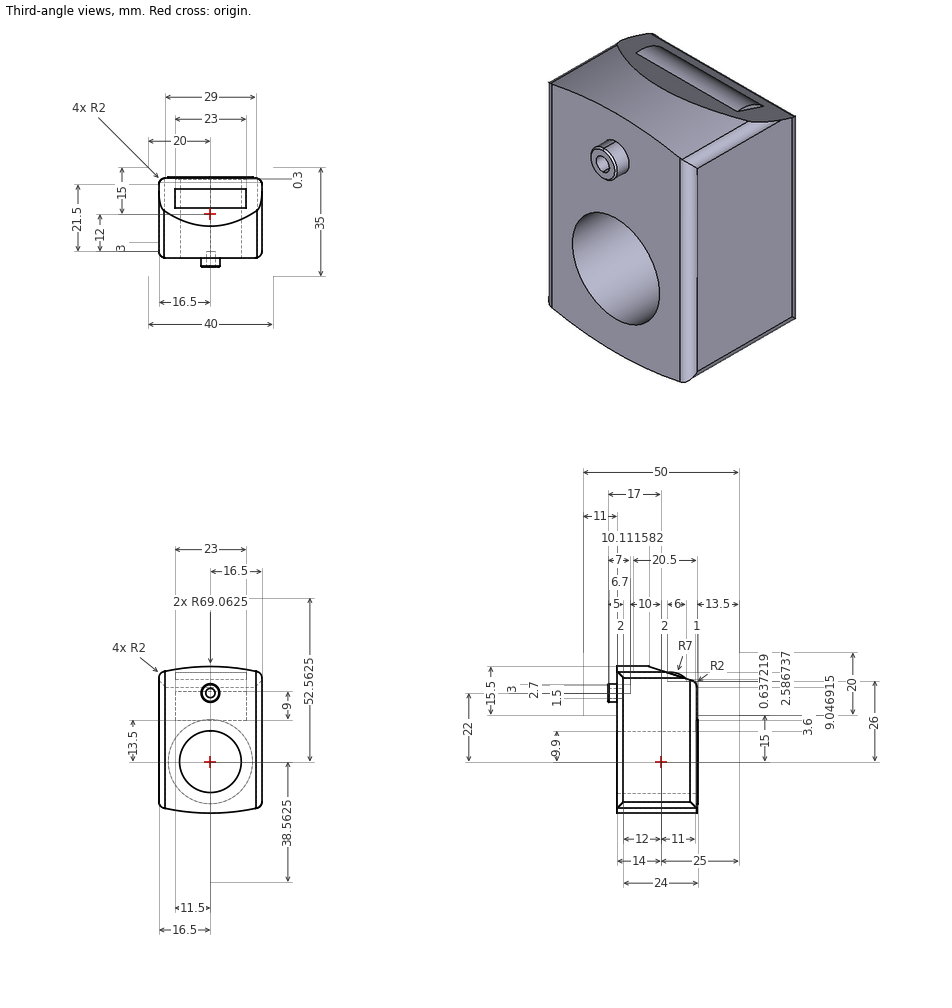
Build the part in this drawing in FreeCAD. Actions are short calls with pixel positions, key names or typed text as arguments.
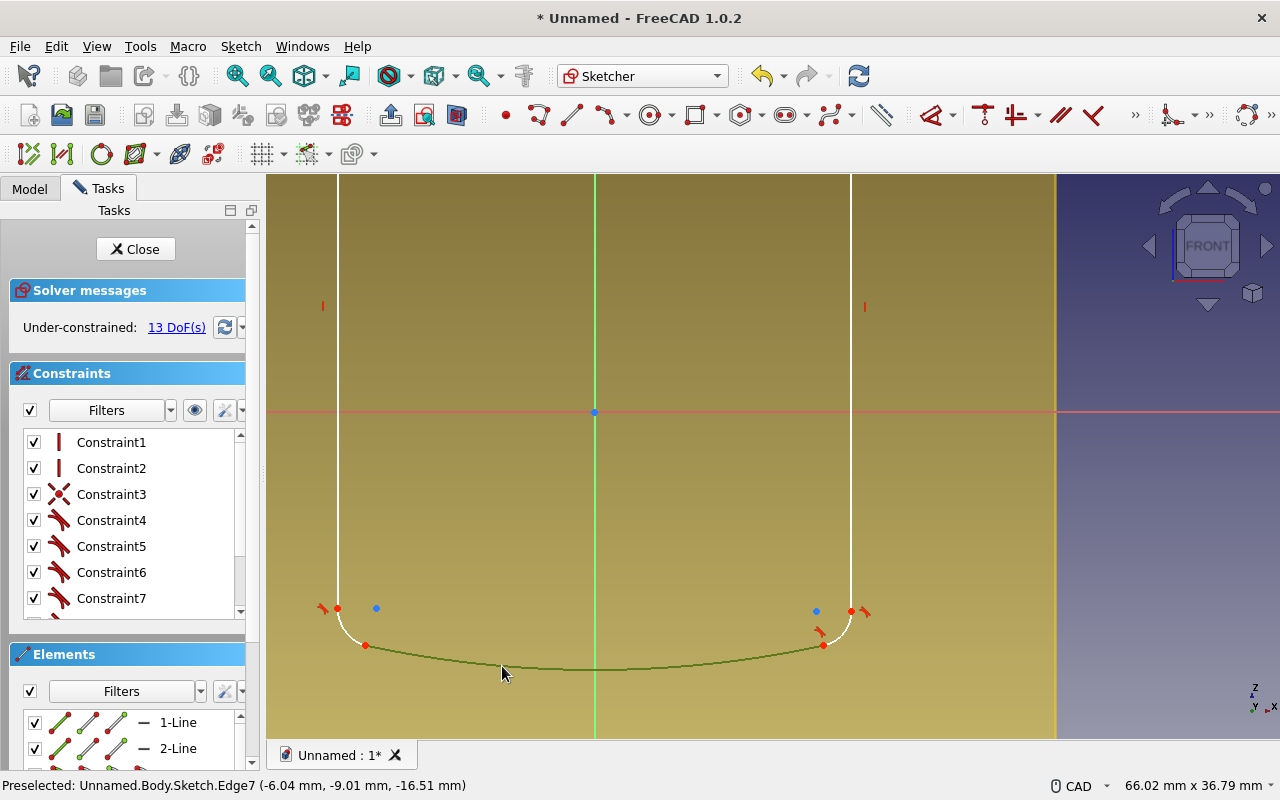
click(341, 623)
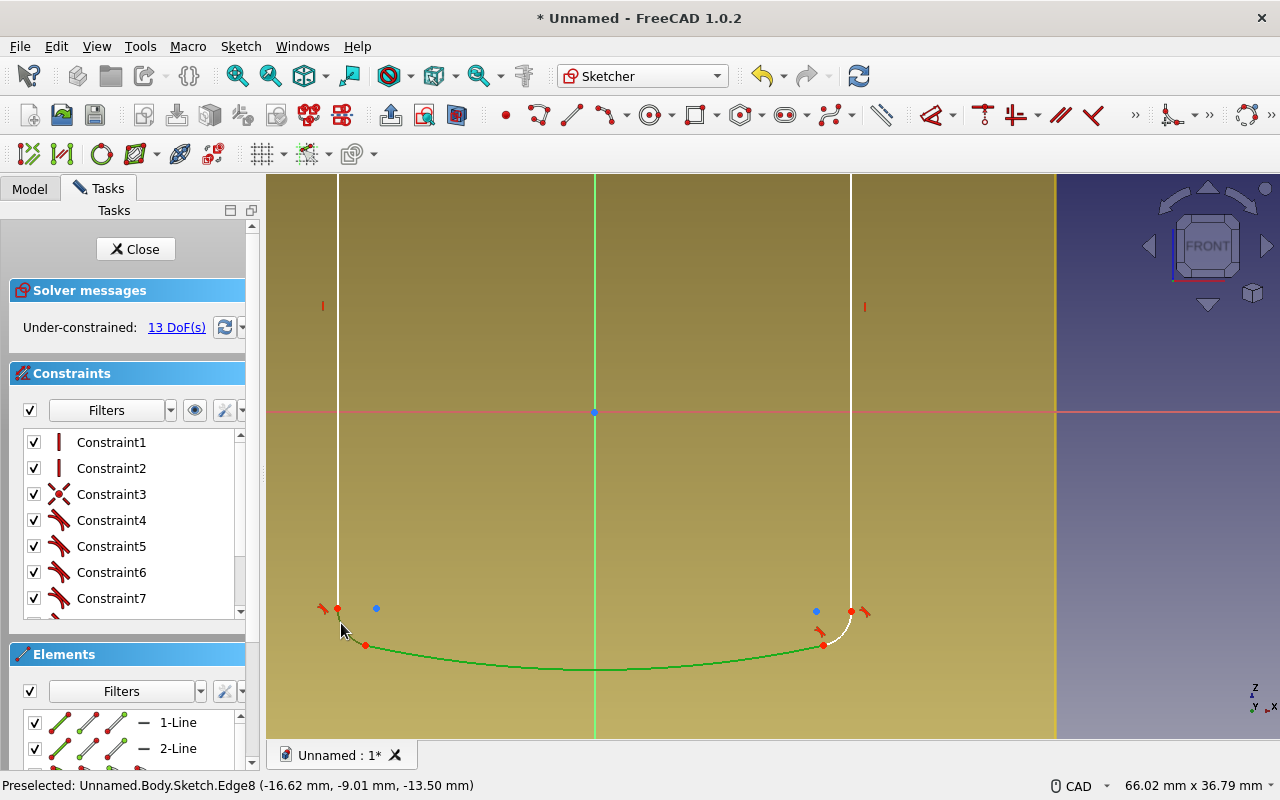
key(t)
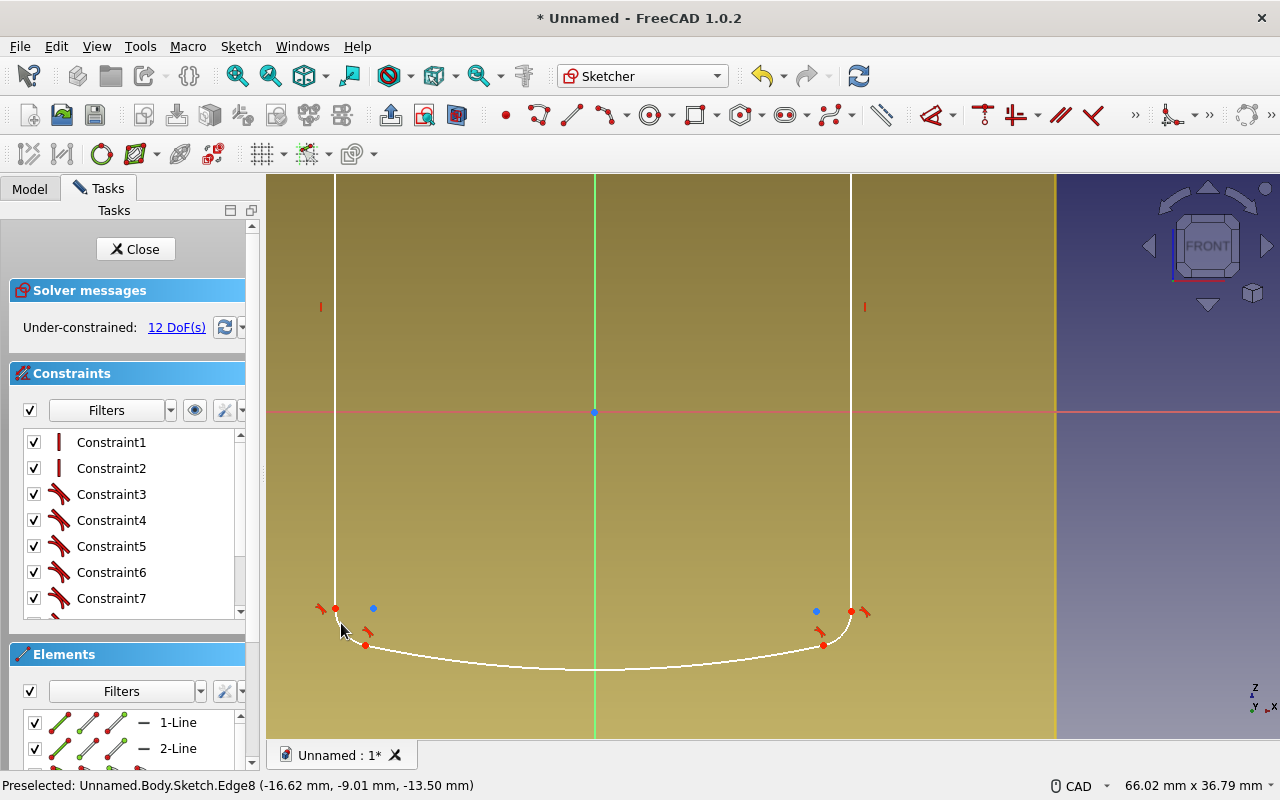
scroll(838, 641, down, 3)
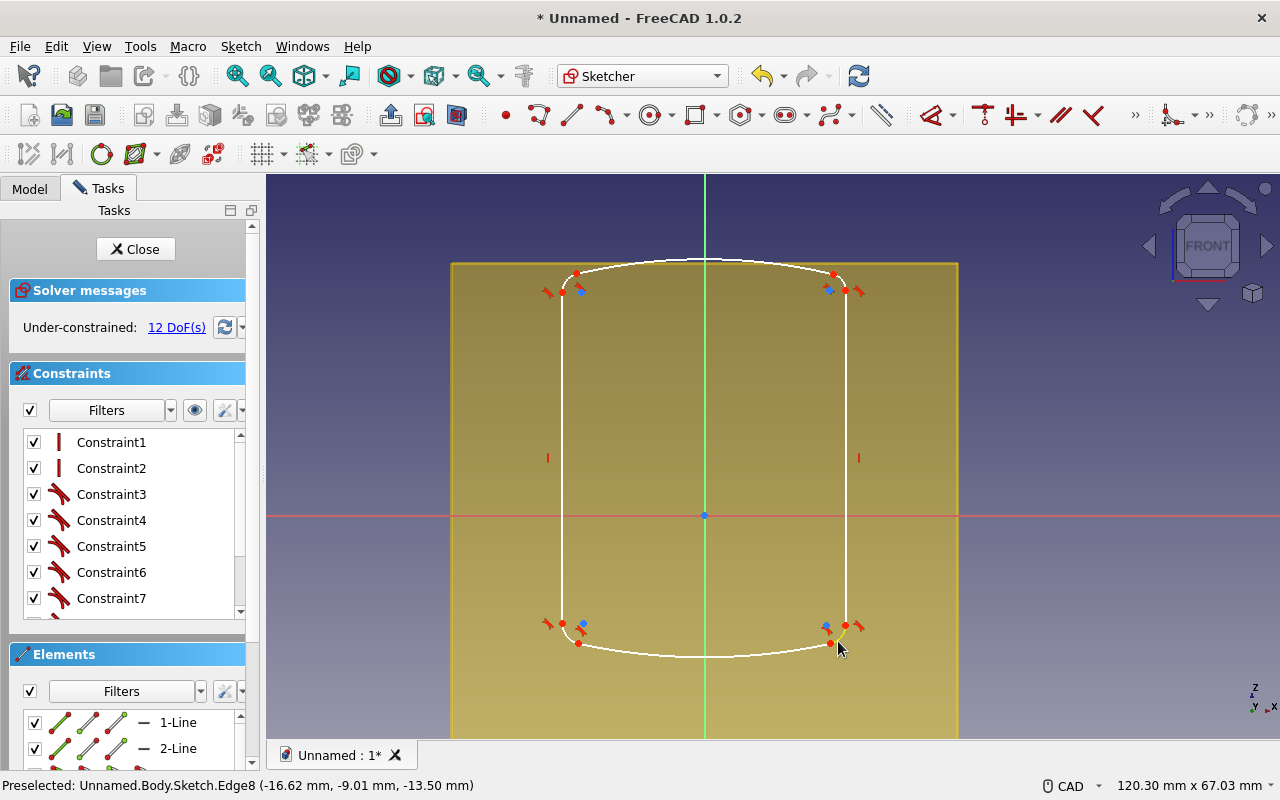
scroll(570, 277, up, 4)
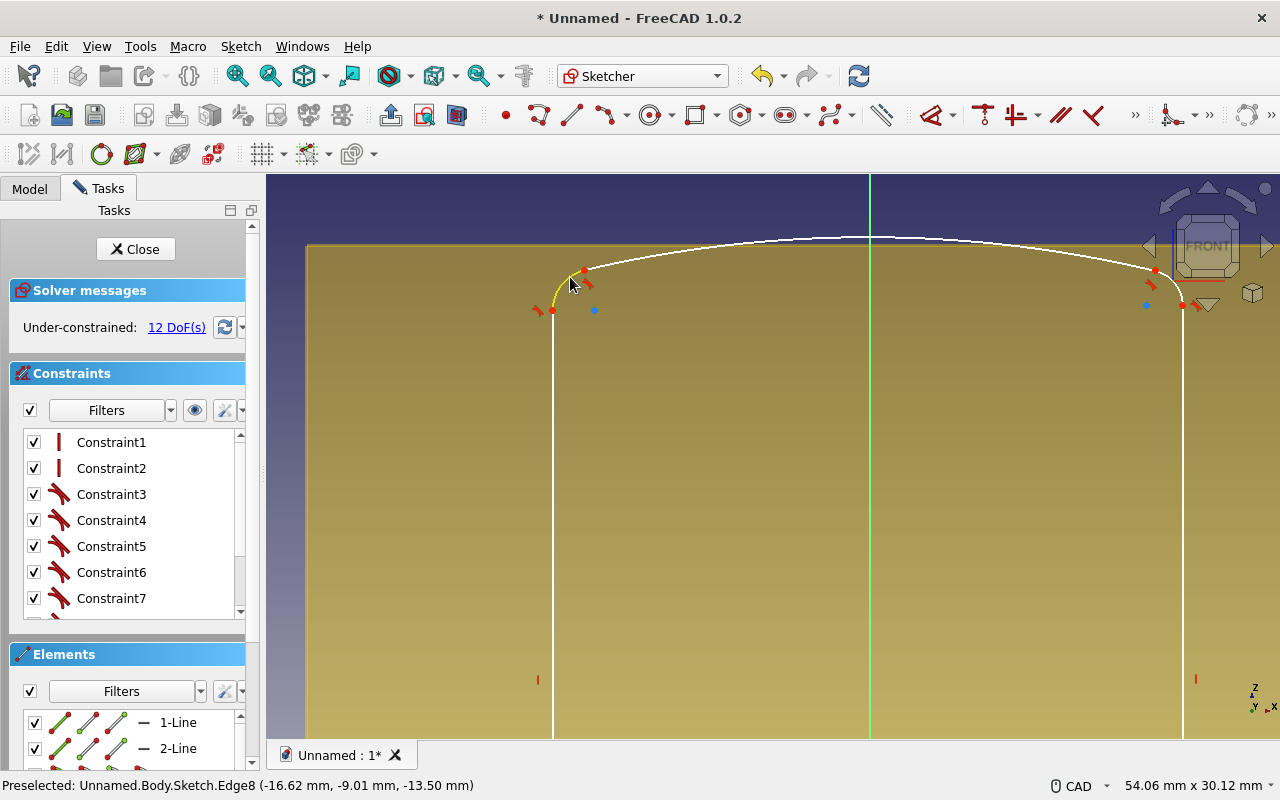
click(570, 277)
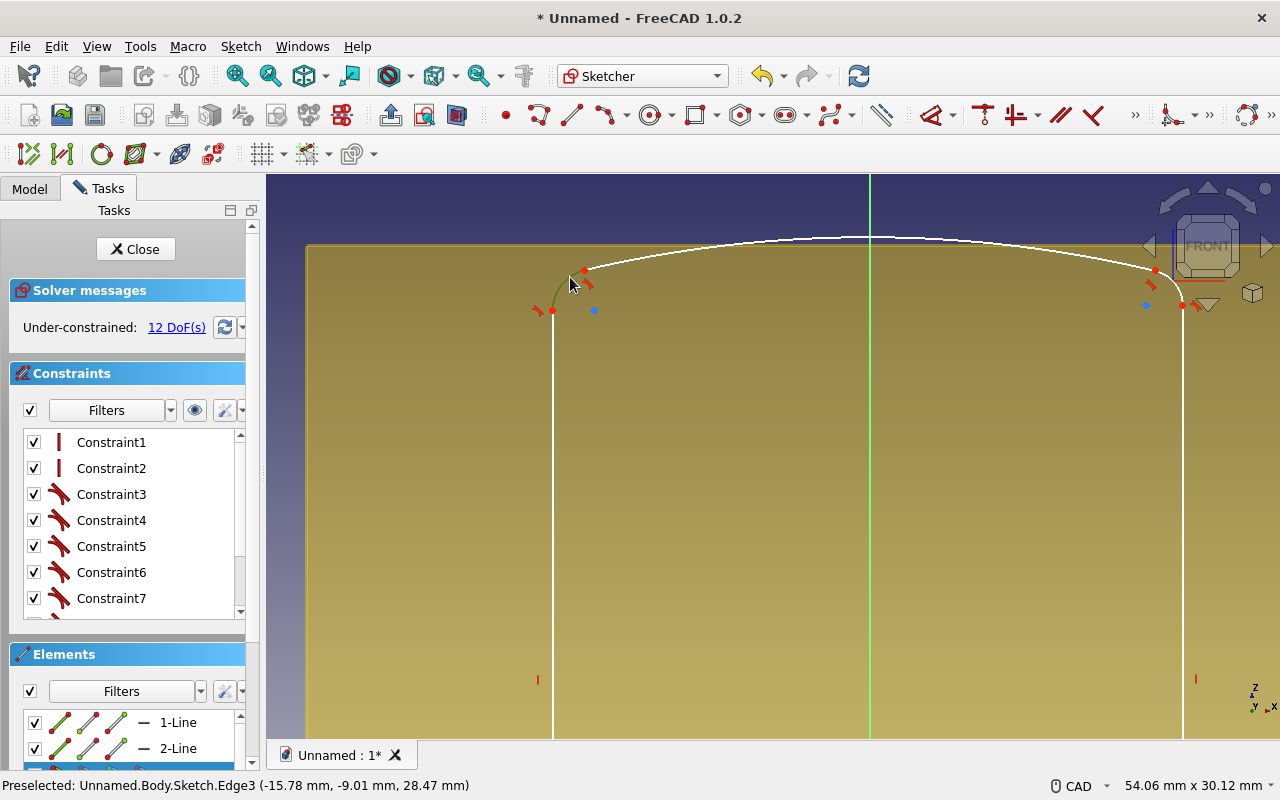
scroll(570, 276, down, 4)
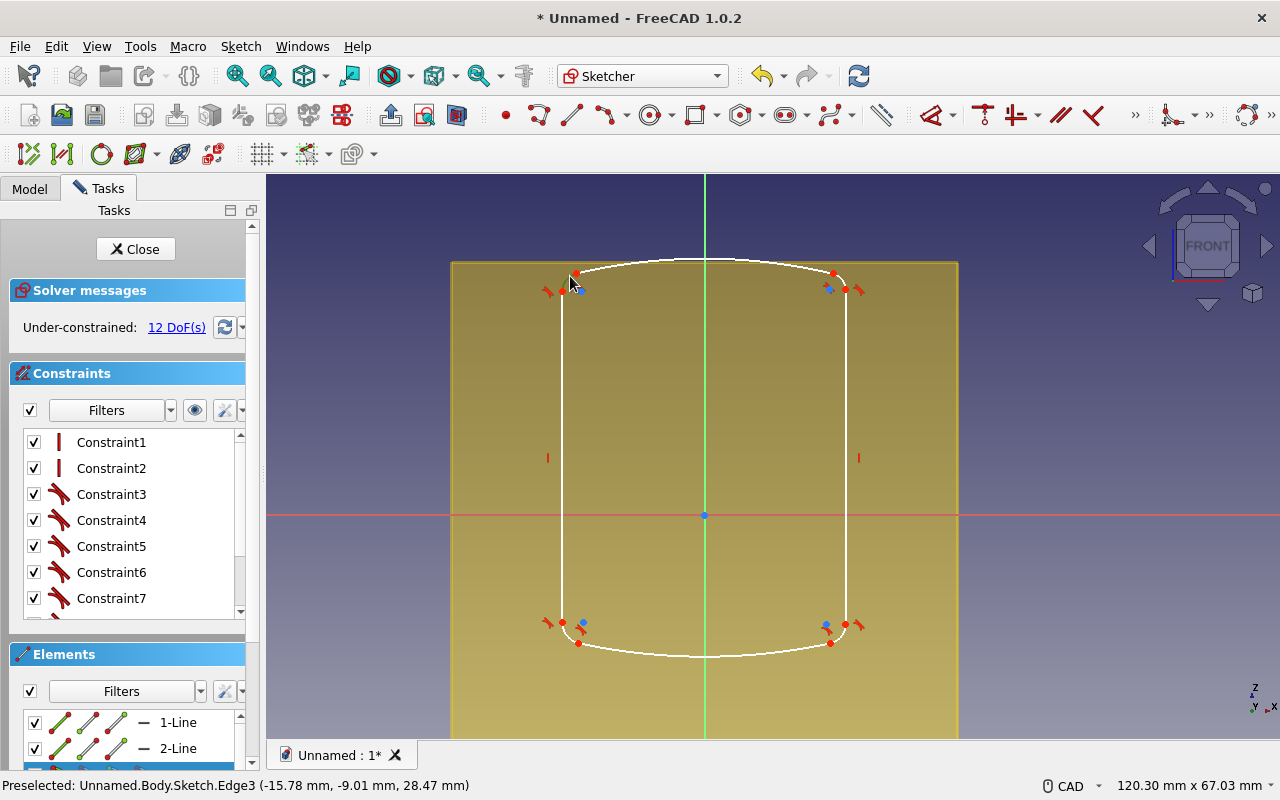
scroll(844, 283, up, 4)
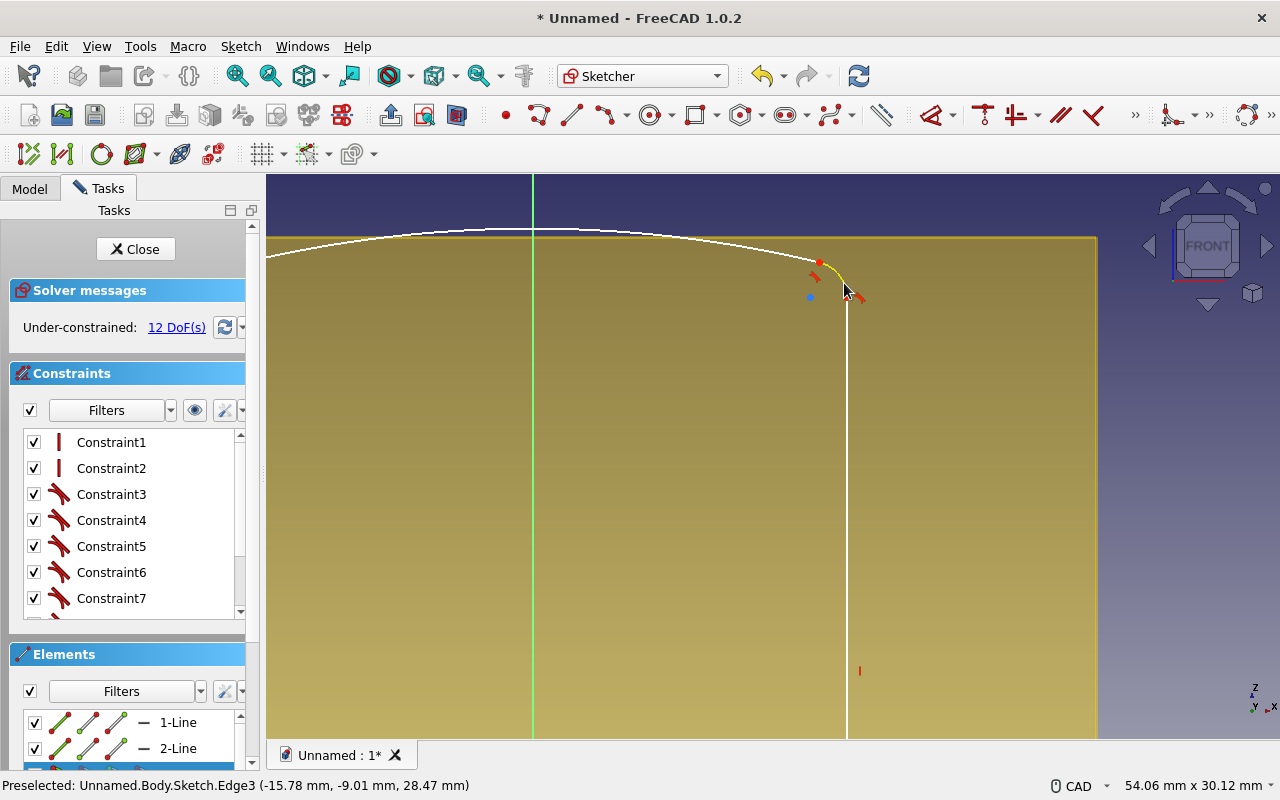
click(844, 283)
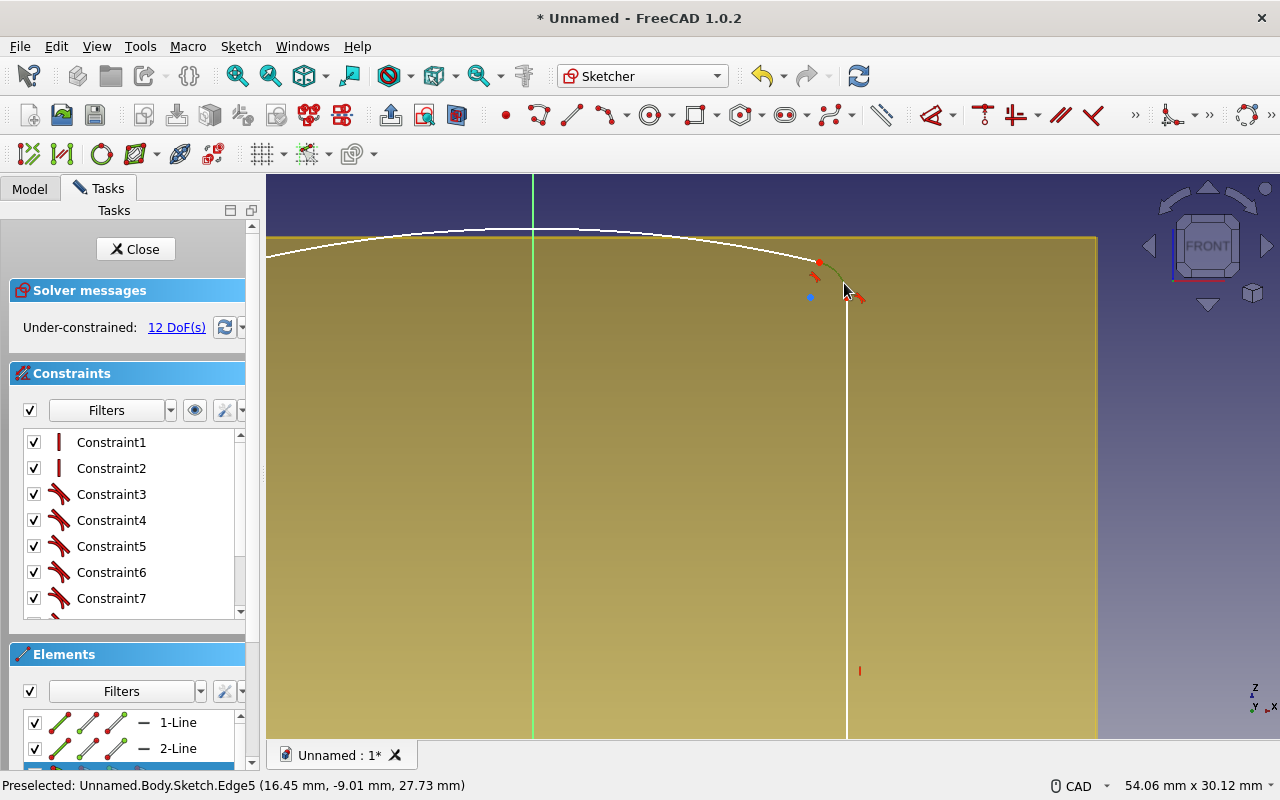
scroll(844, 283, down, 4)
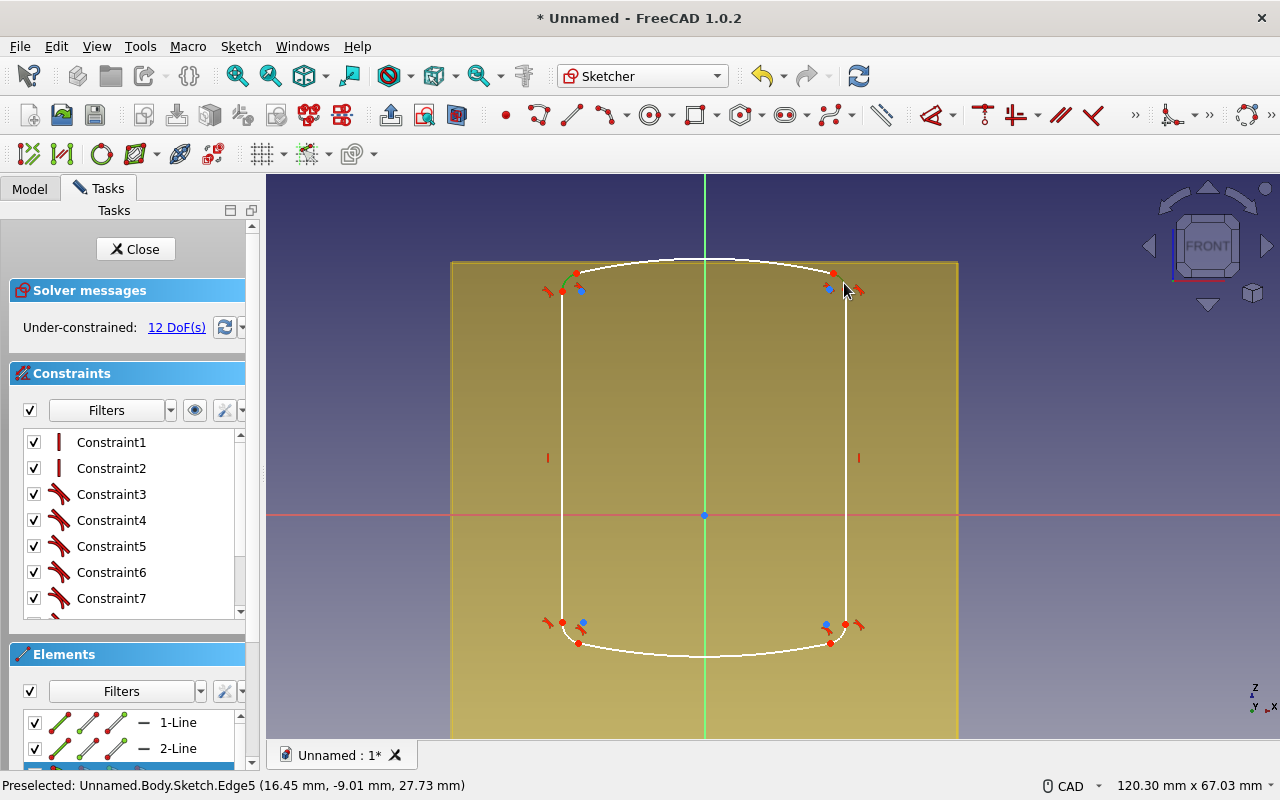
scroll(838, 640, up, 3)